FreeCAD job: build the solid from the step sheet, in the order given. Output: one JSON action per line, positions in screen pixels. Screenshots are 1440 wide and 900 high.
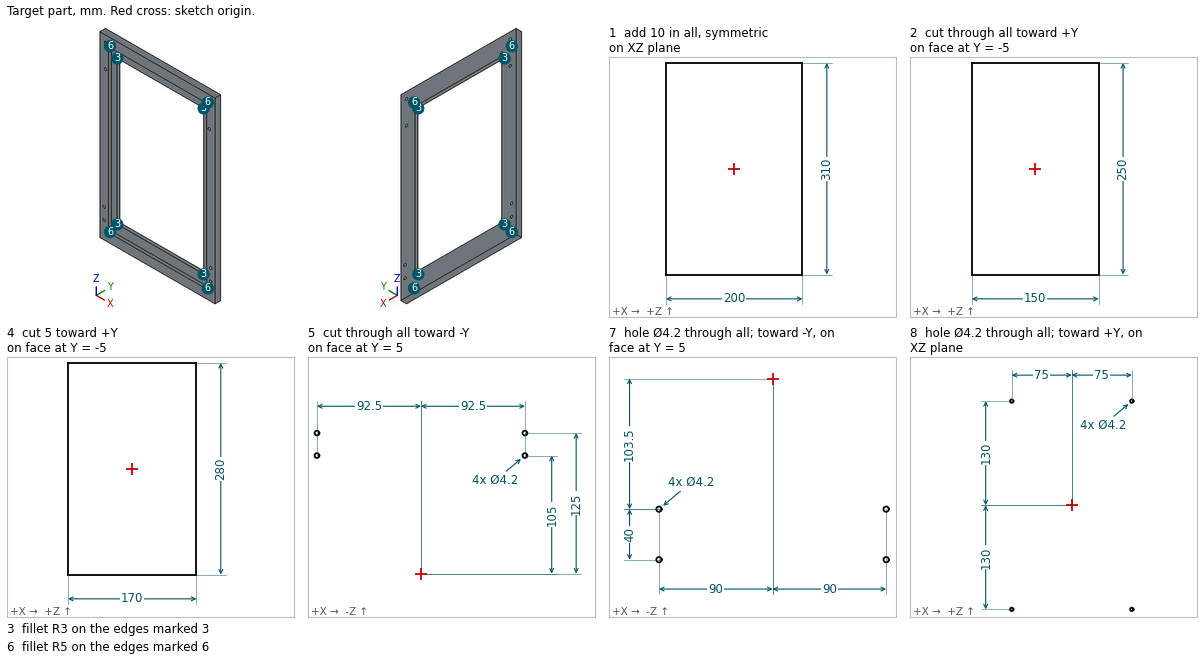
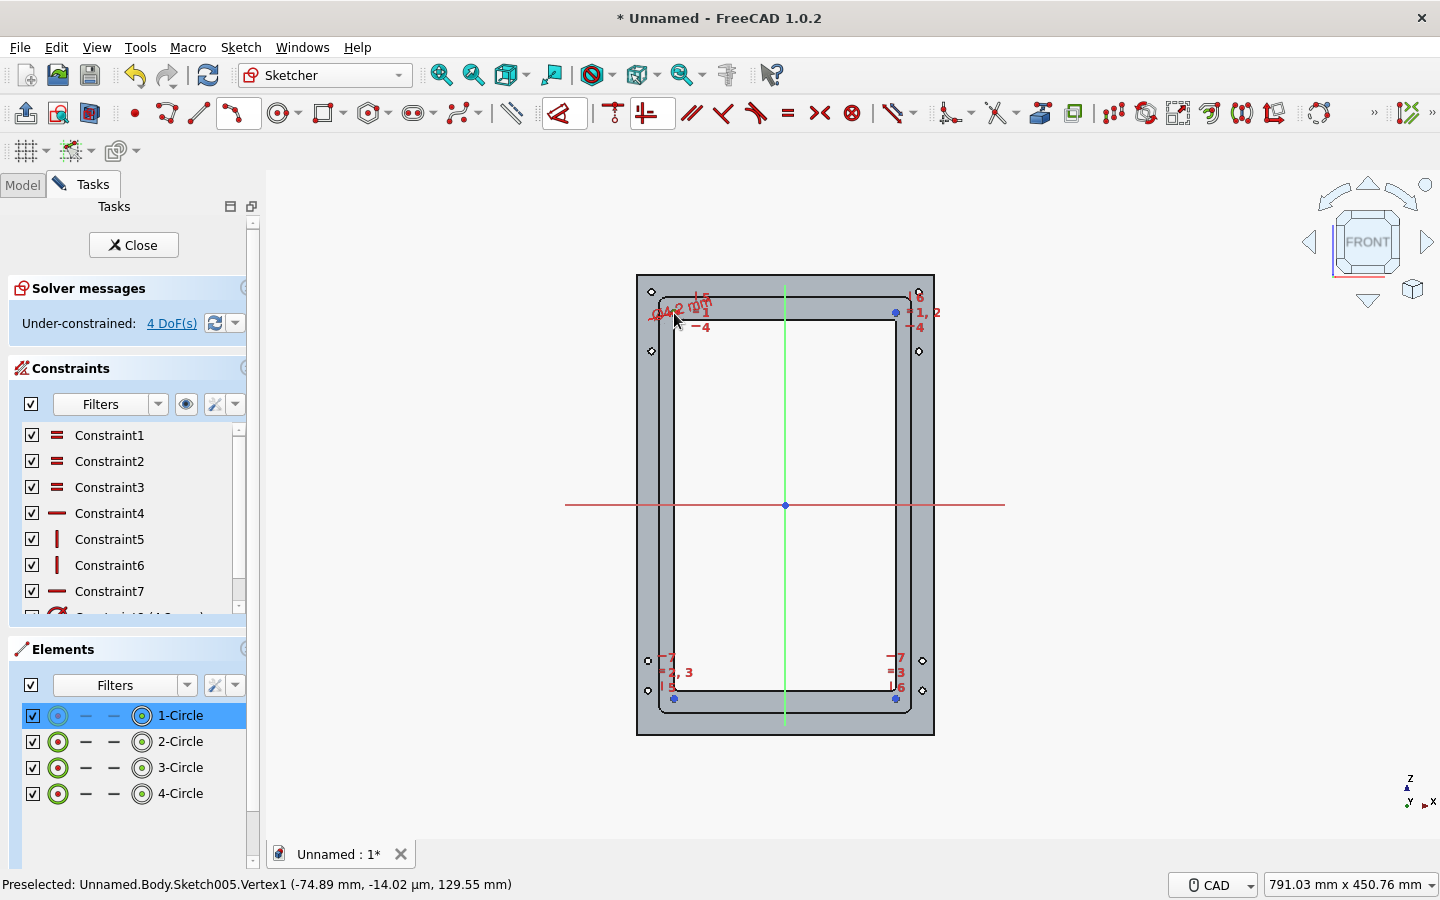
{"action": "key", "text": "l"}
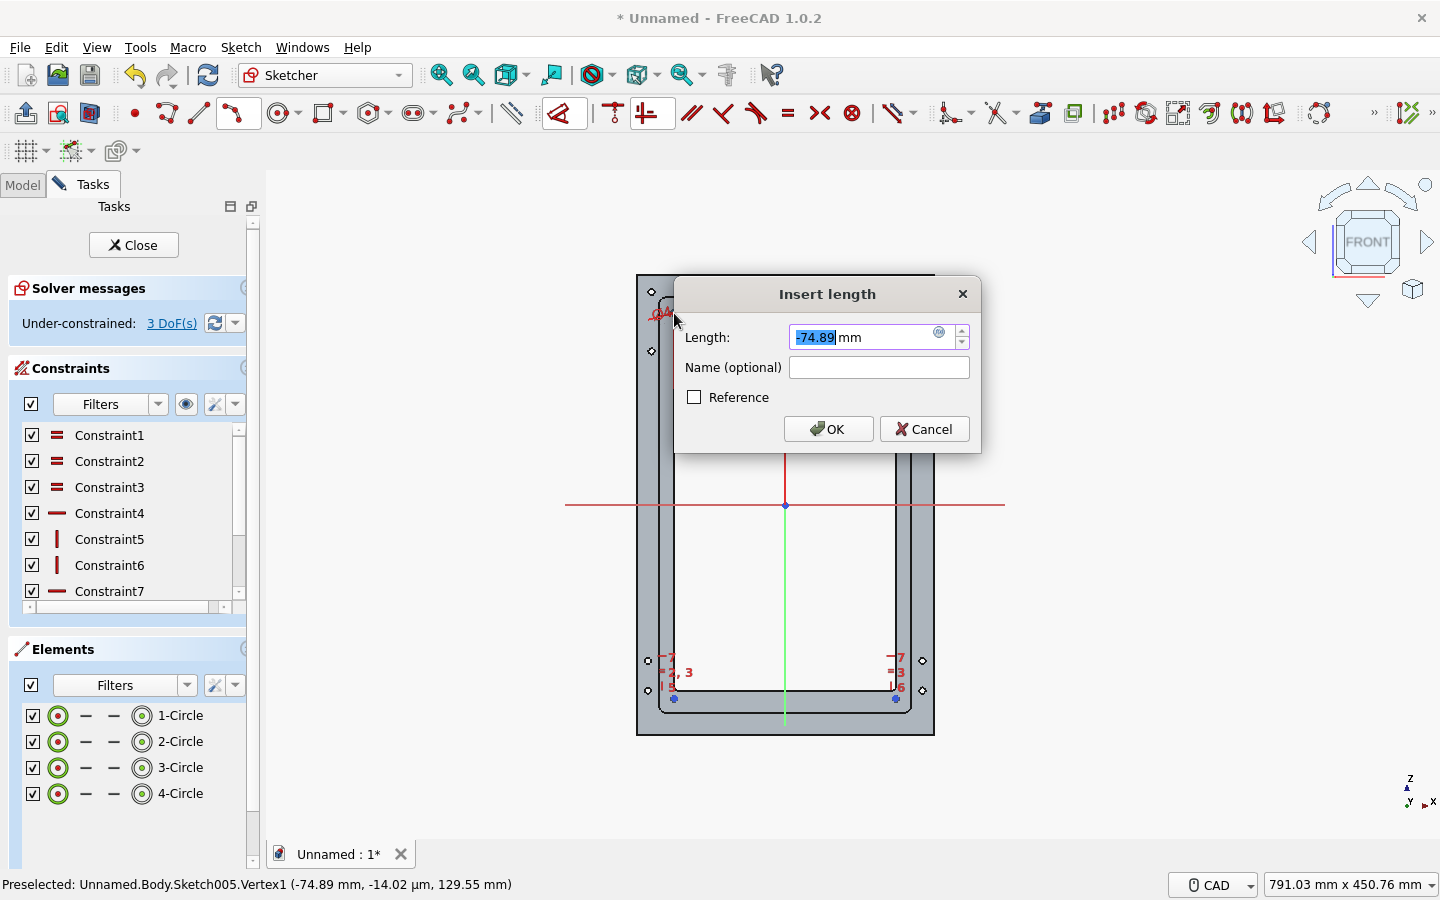
{"action": "type", "text": "-75"}
{"action": "key", "text": "Return"}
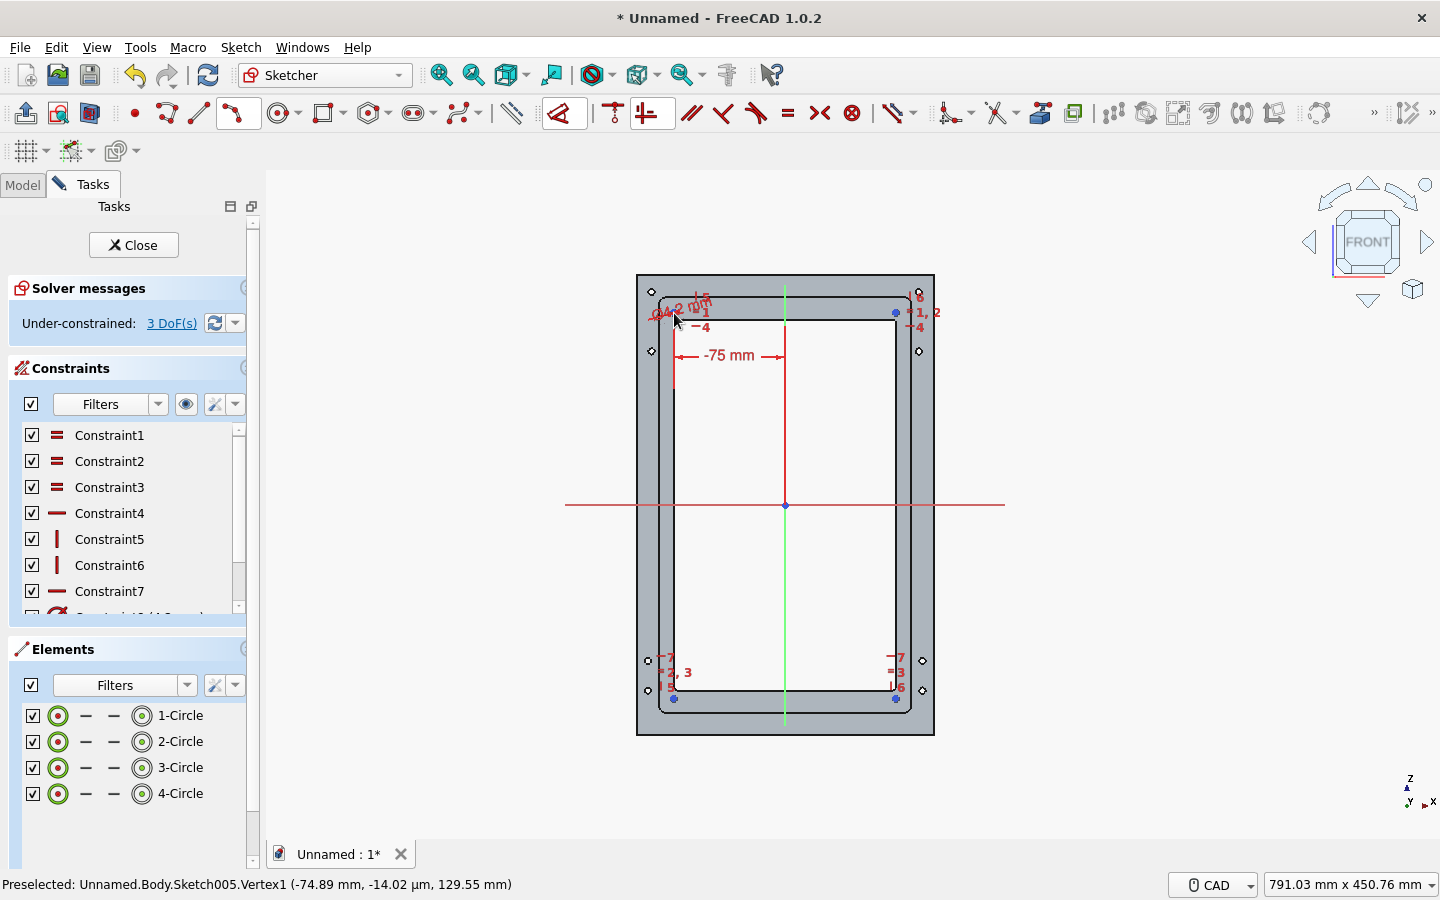
{"action": "left_click", "coordinate": [896, 313]}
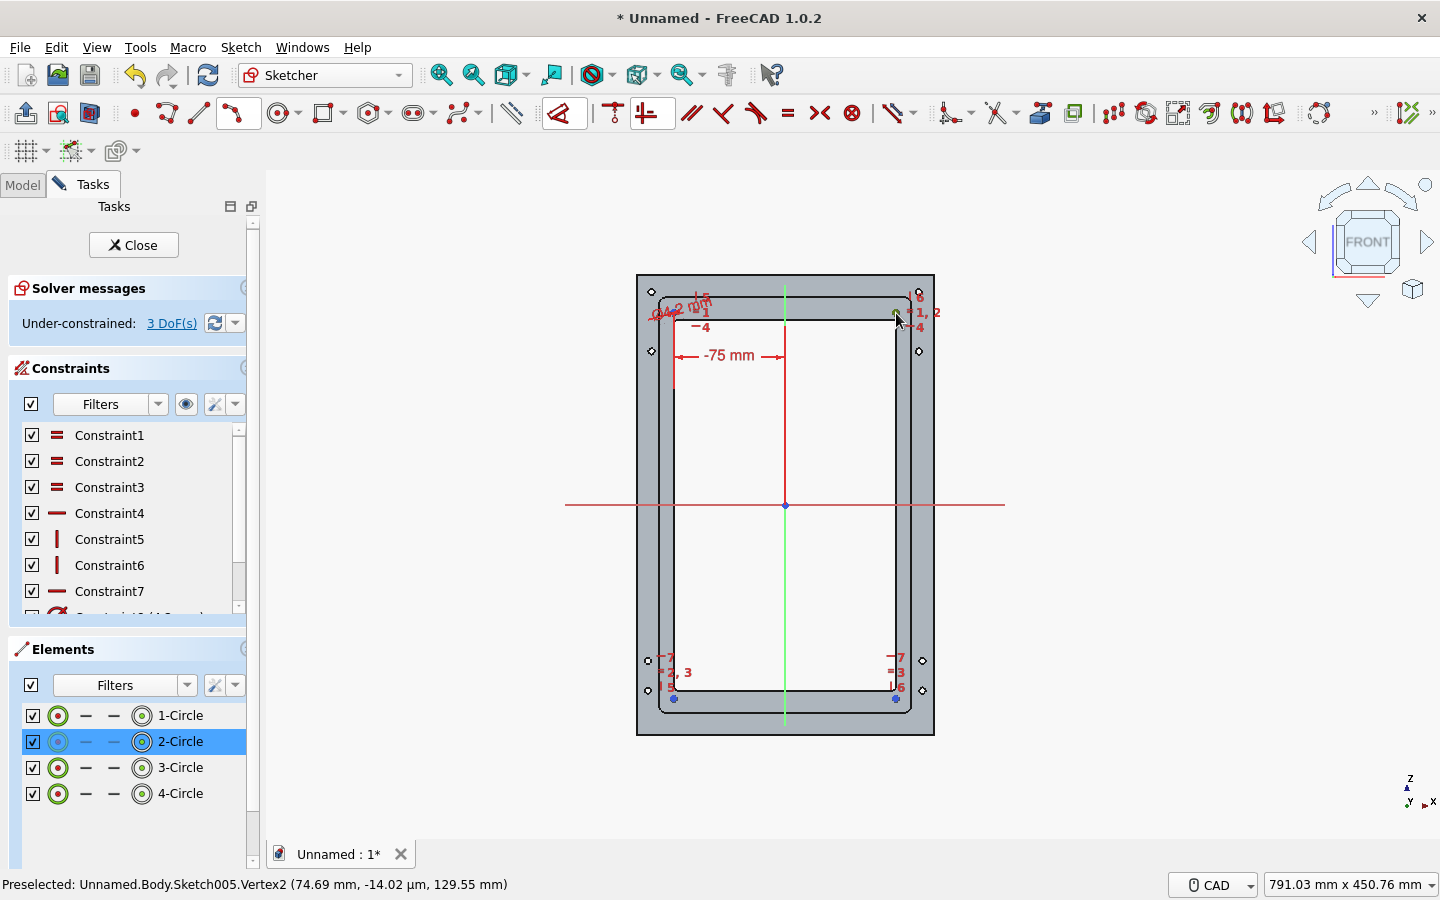
{"action": "key", "text": "l"}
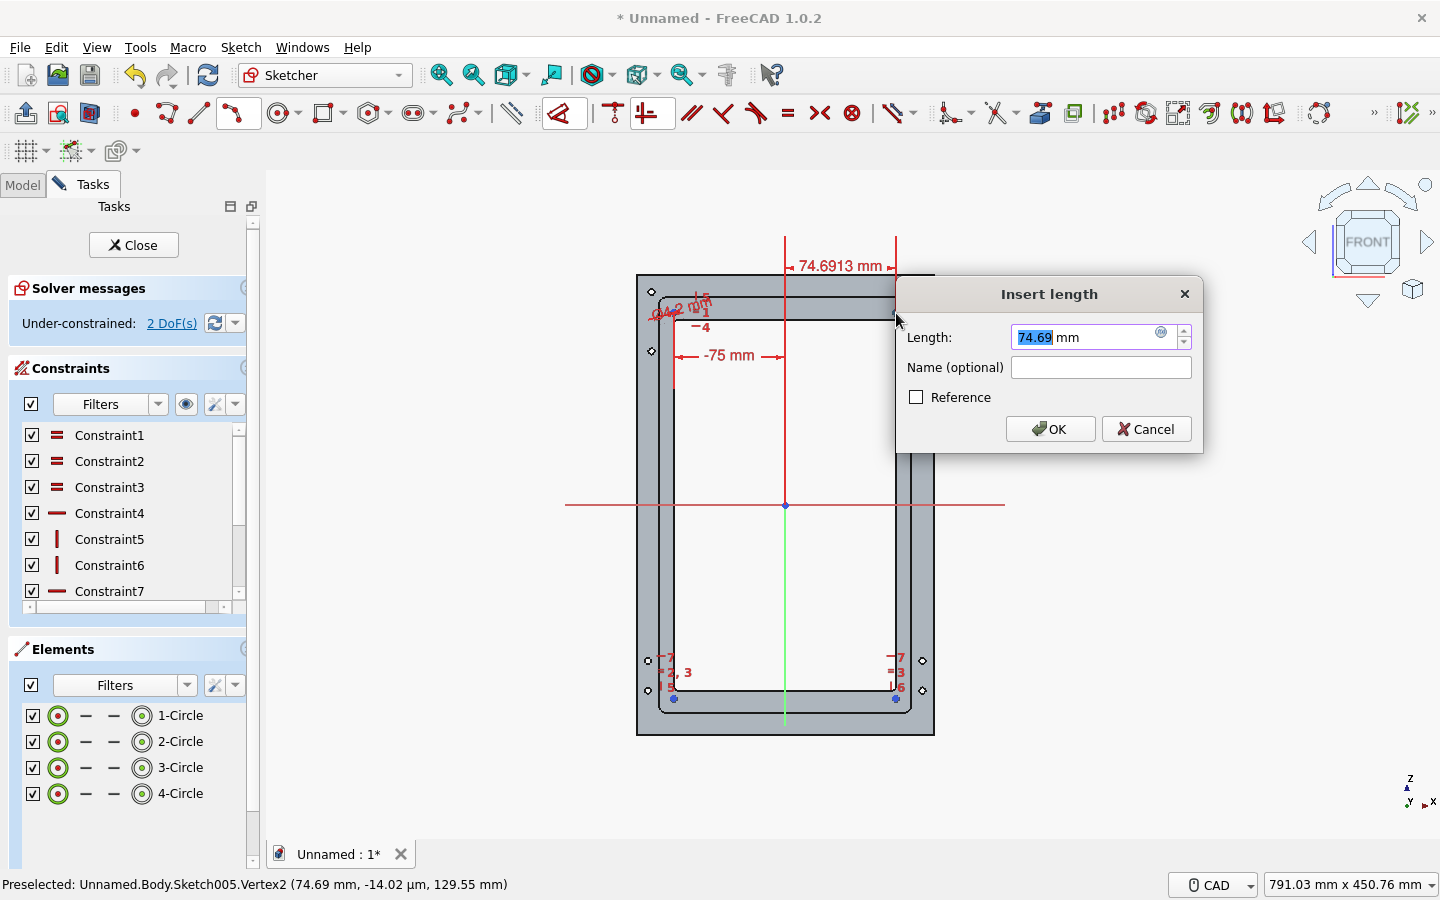
{"action": "type", "text": "75"}
{"action": "key", "text": "Return"}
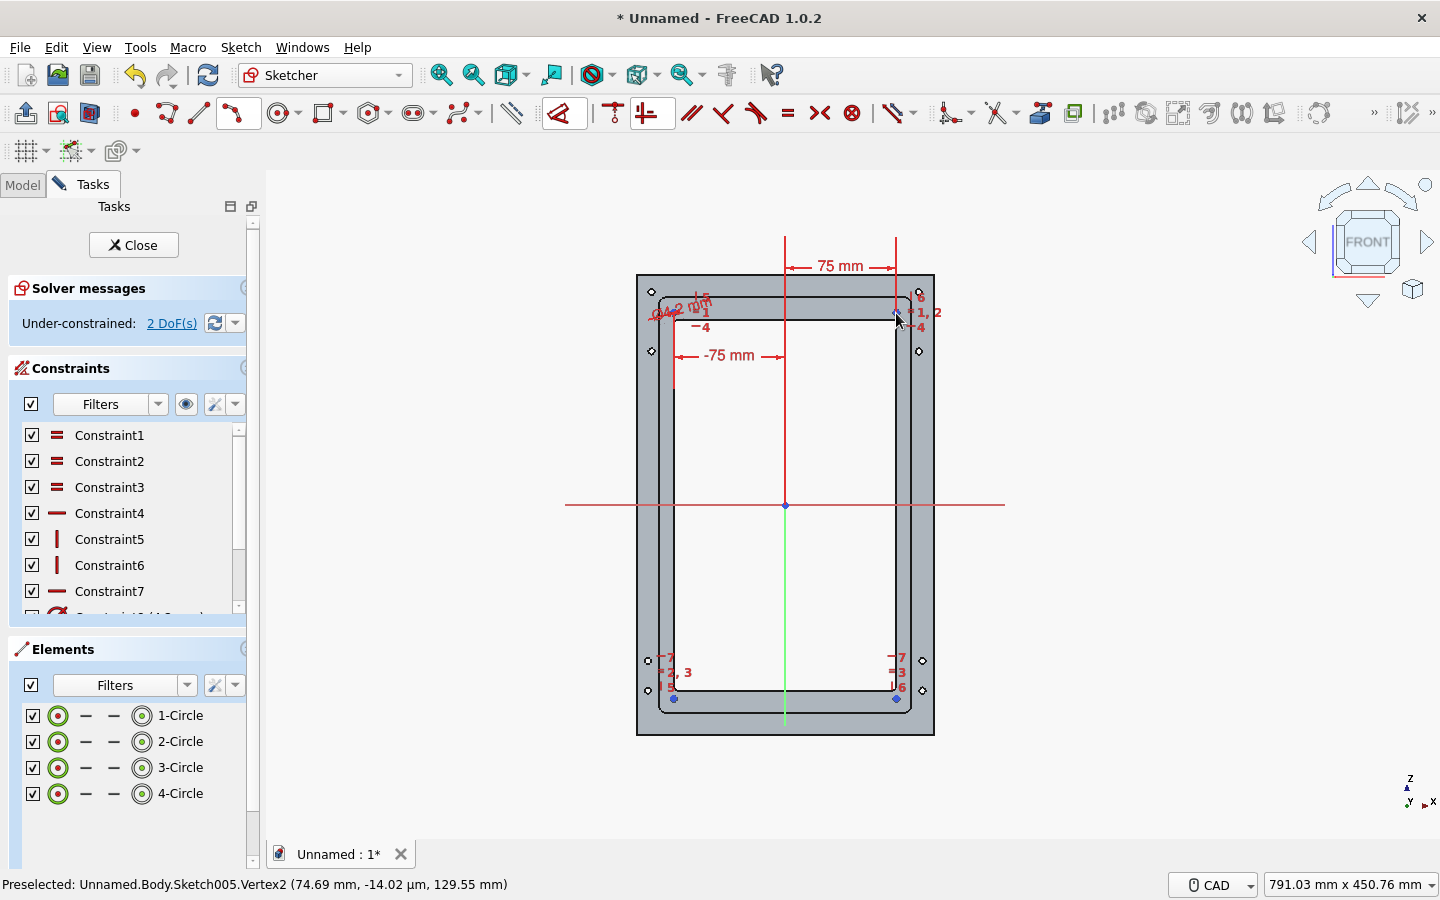
{"action": "left_click", "coordinate": [674, 313]}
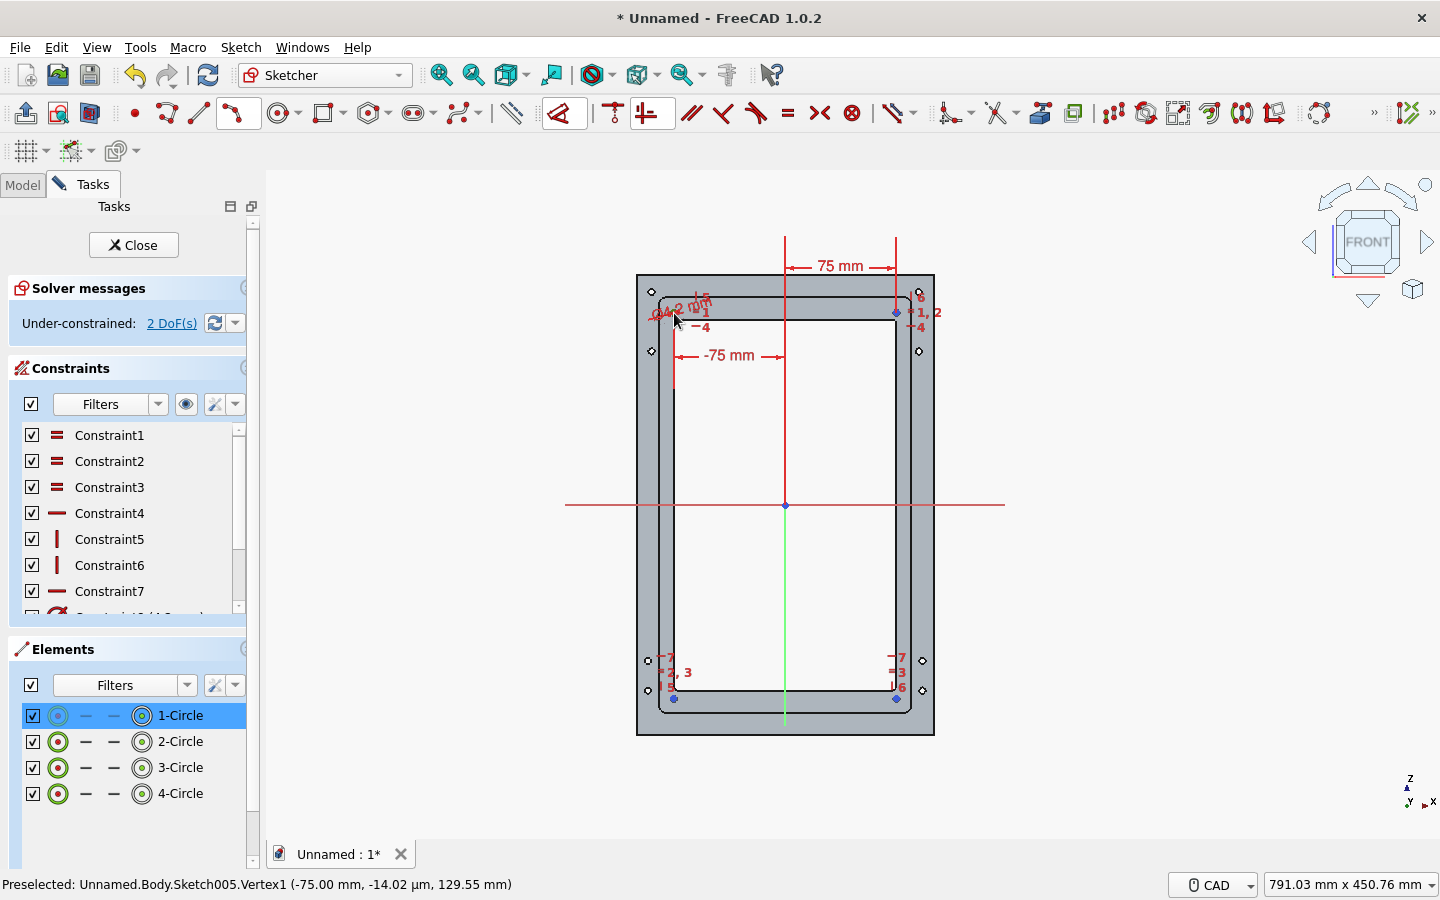
{"action": "key", "text": "i"}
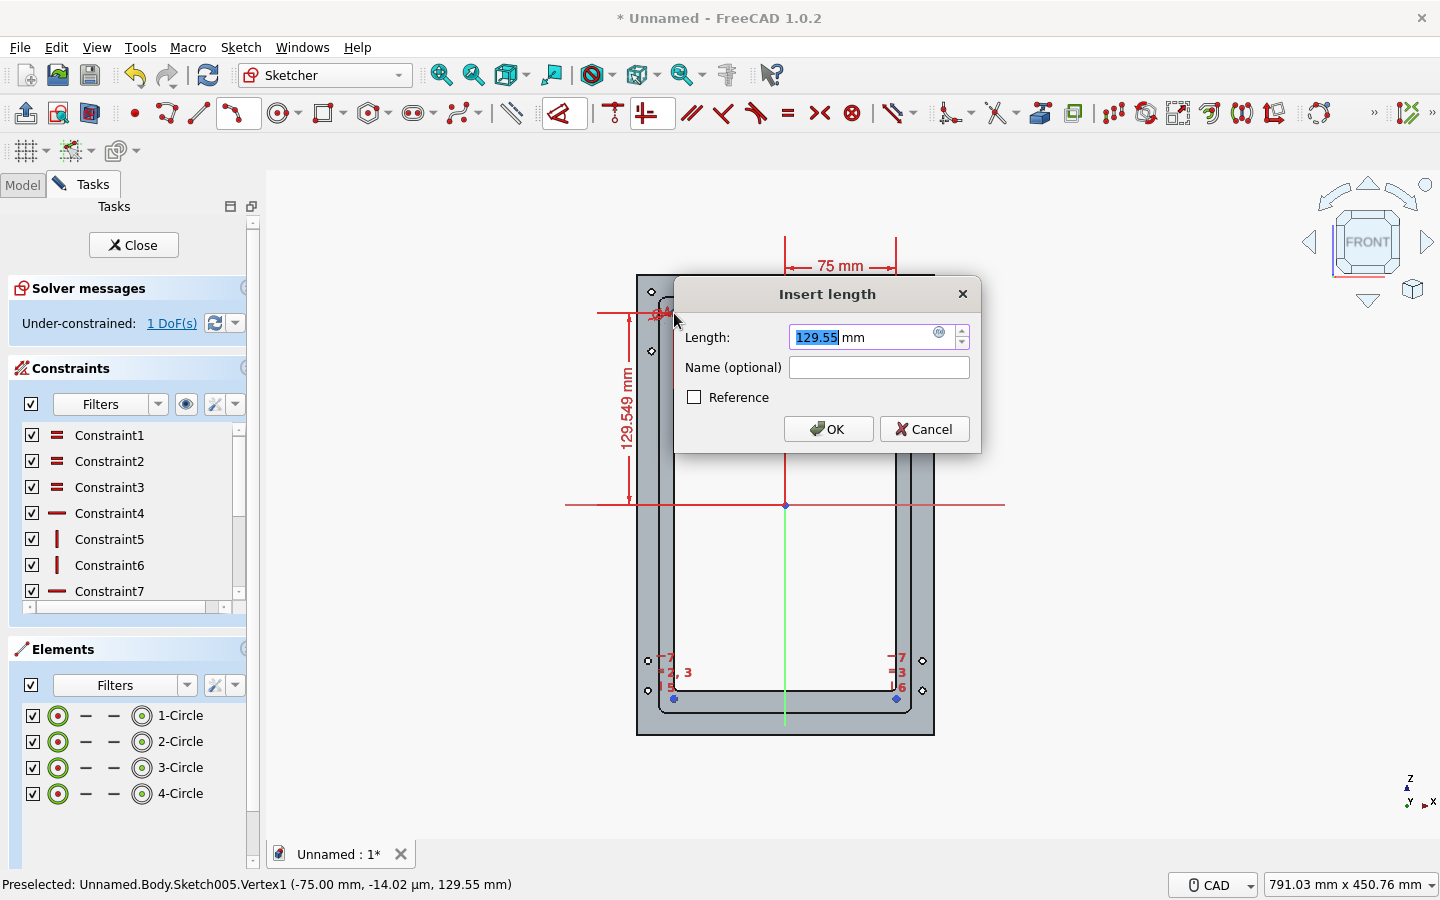
{"action": "type", "text": "130"}
{"action": "key", "text": "Return"}